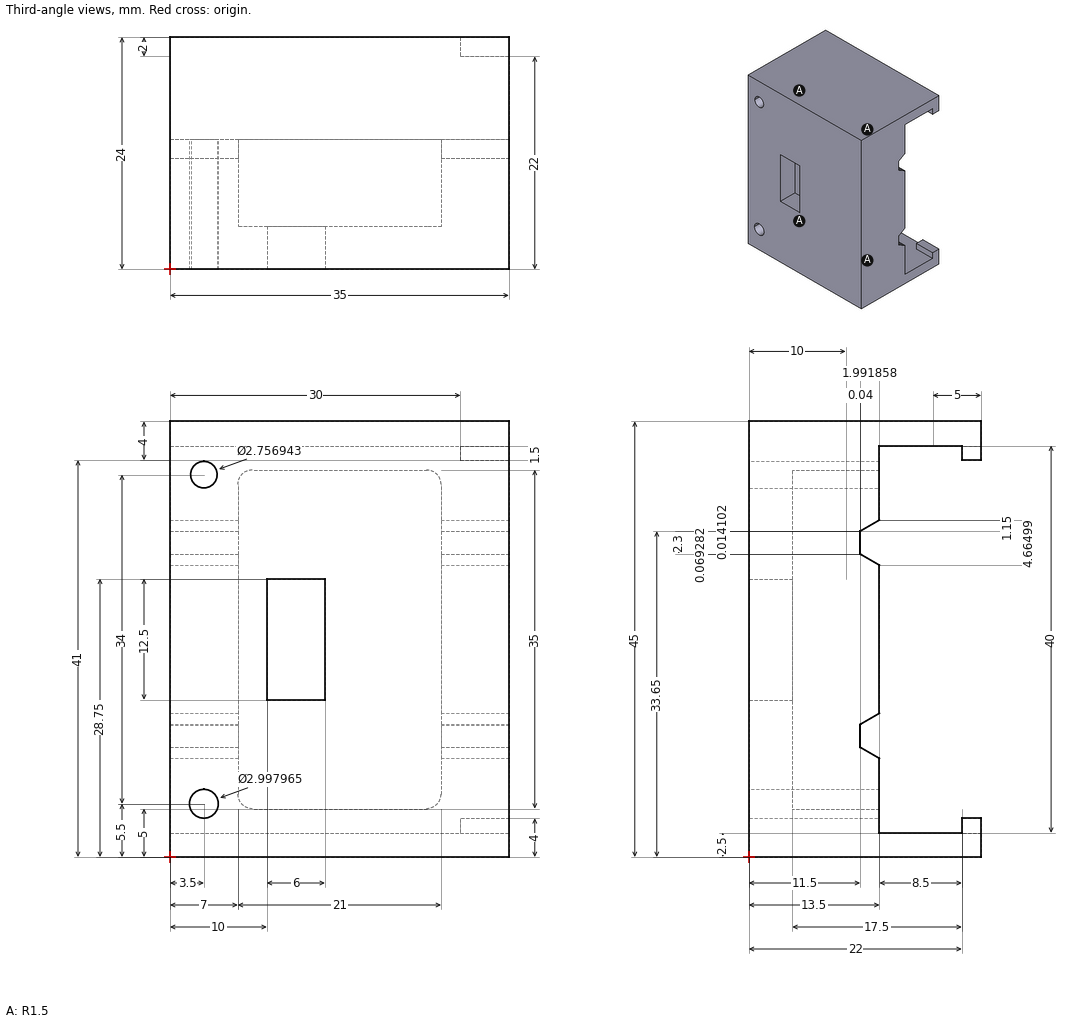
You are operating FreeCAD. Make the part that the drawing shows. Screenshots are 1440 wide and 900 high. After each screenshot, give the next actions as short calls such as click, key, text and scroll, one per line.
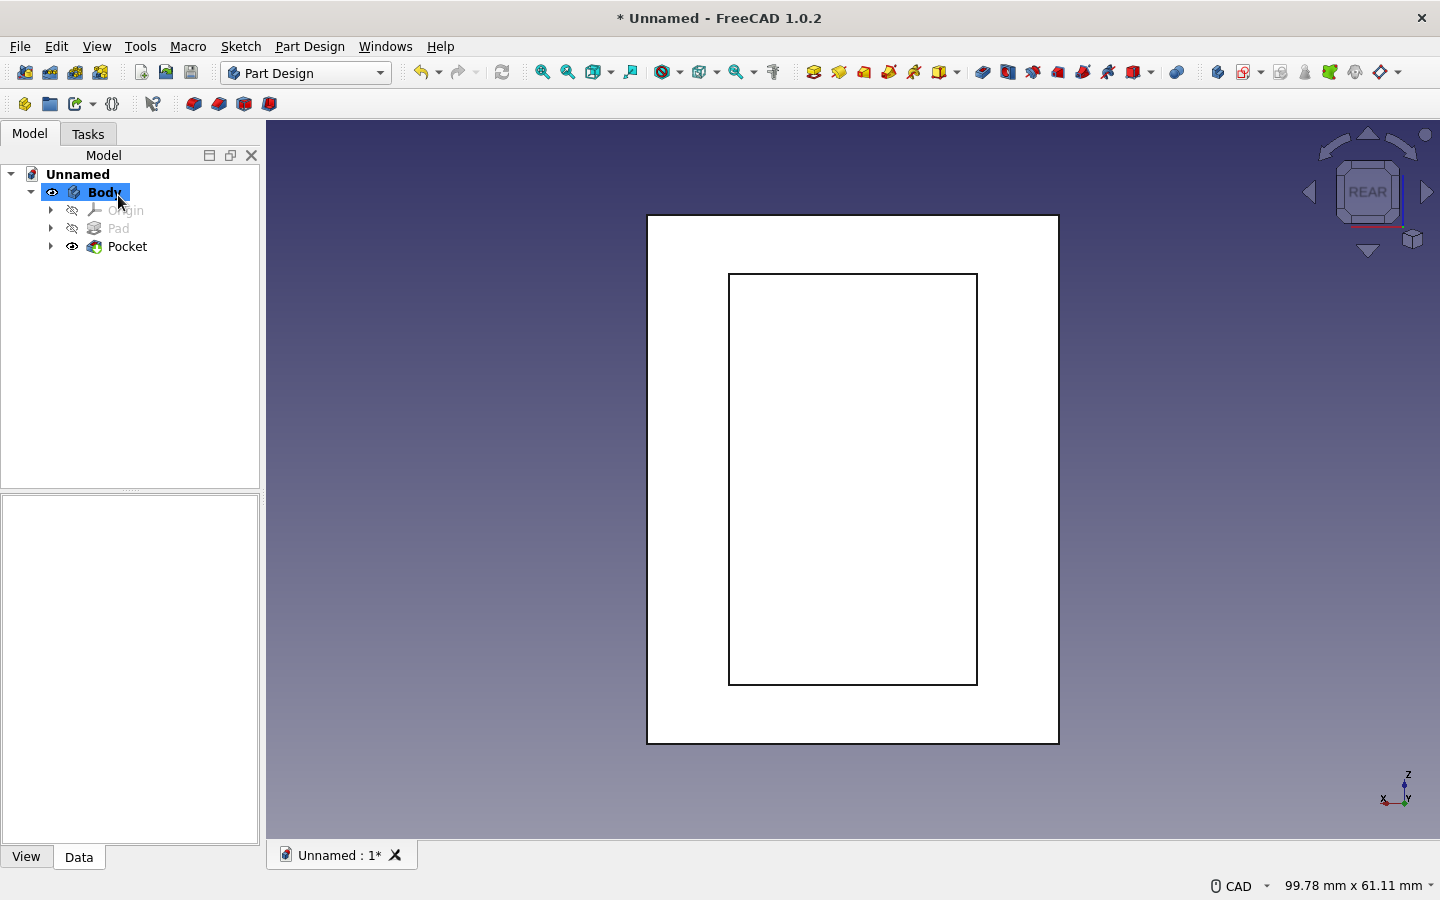
click(1242, 72)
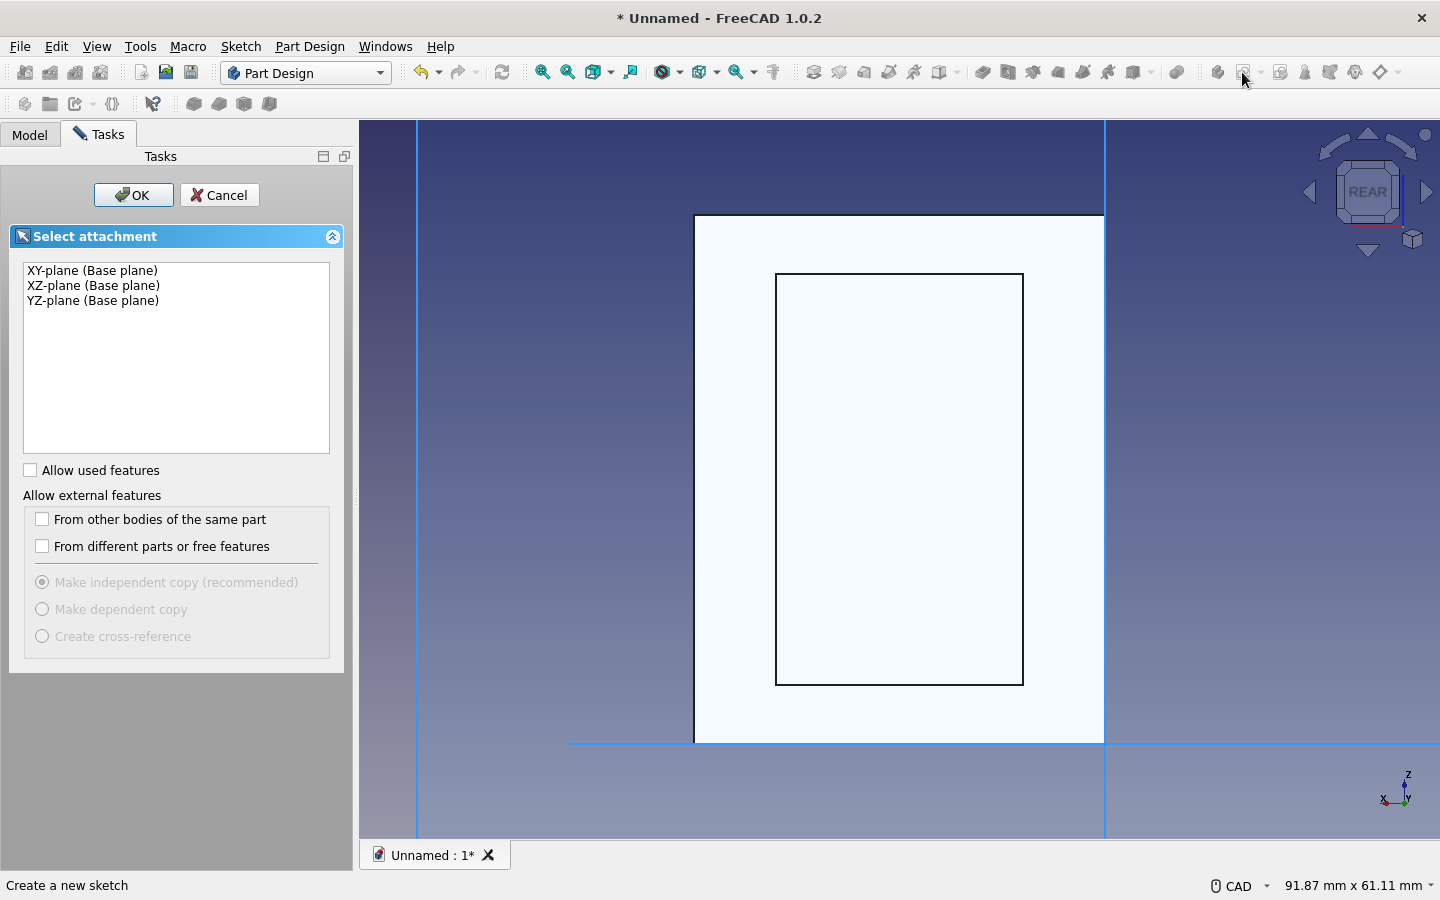
click(84, 300)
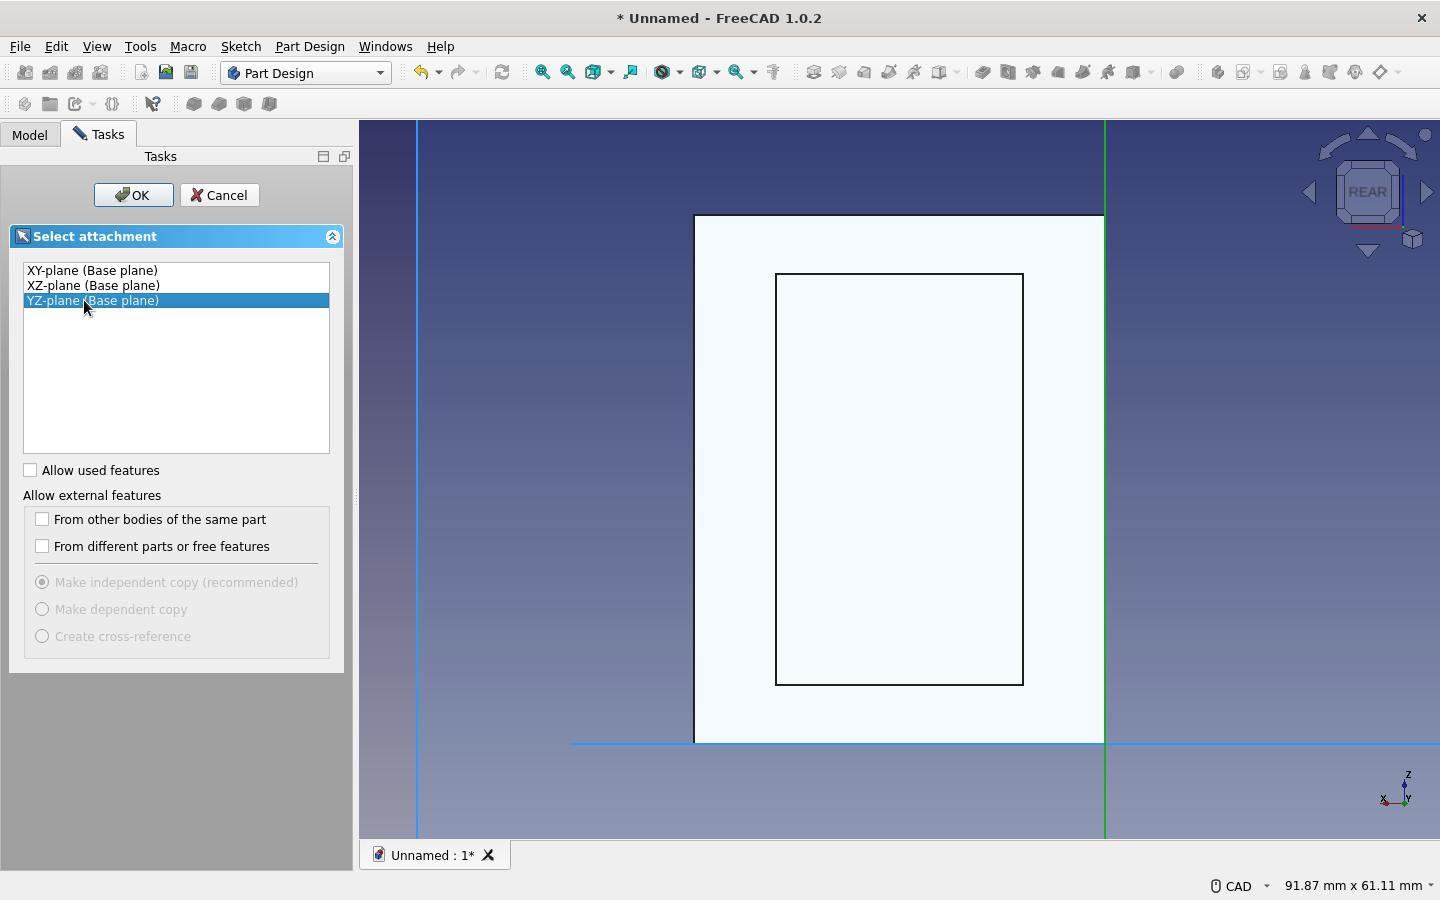
click(134, 195)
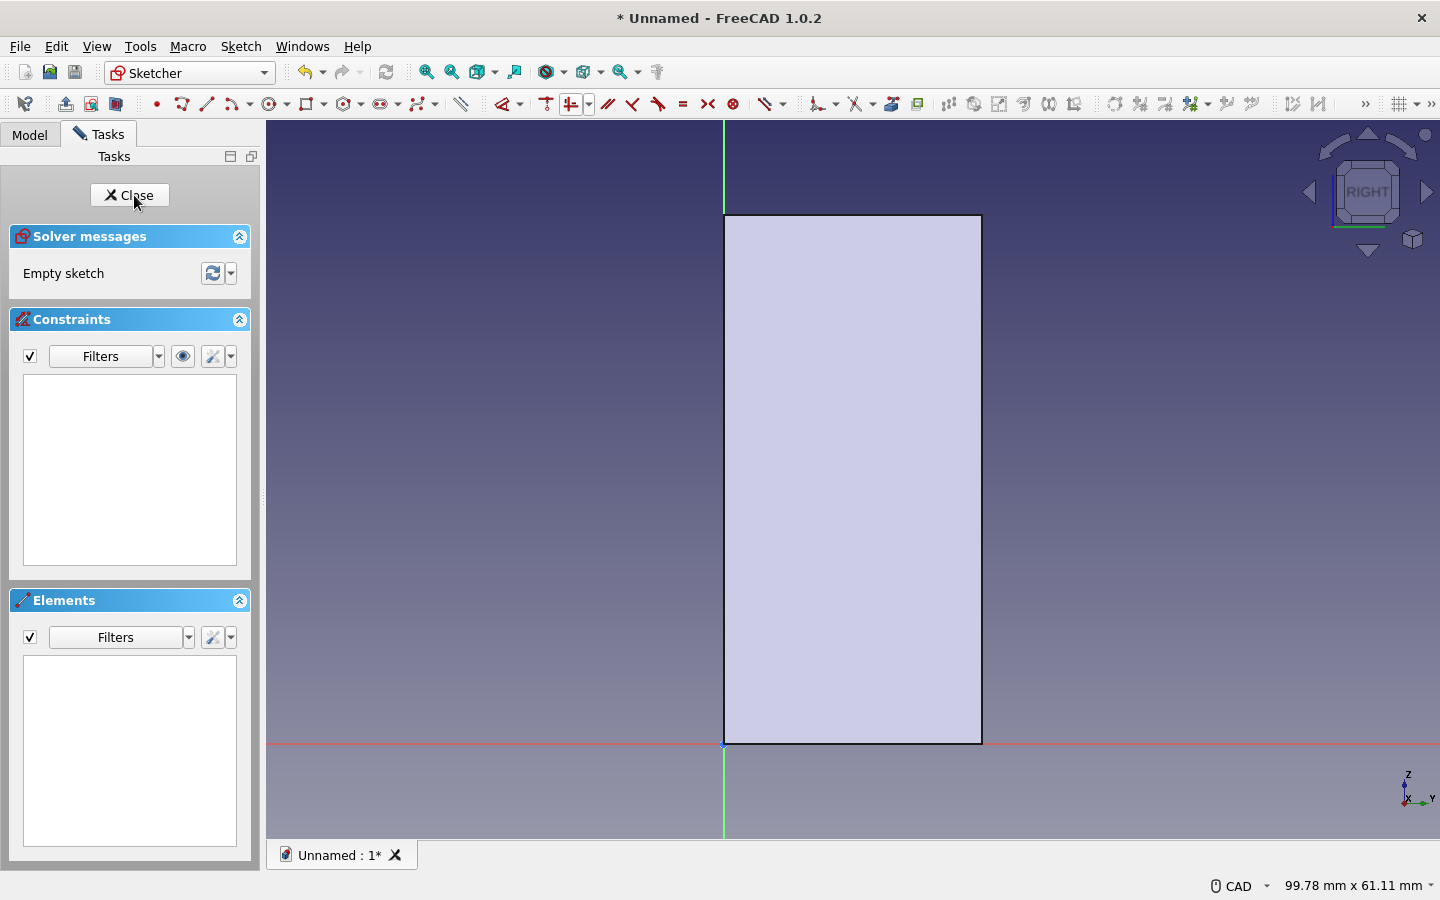
click(116, 104)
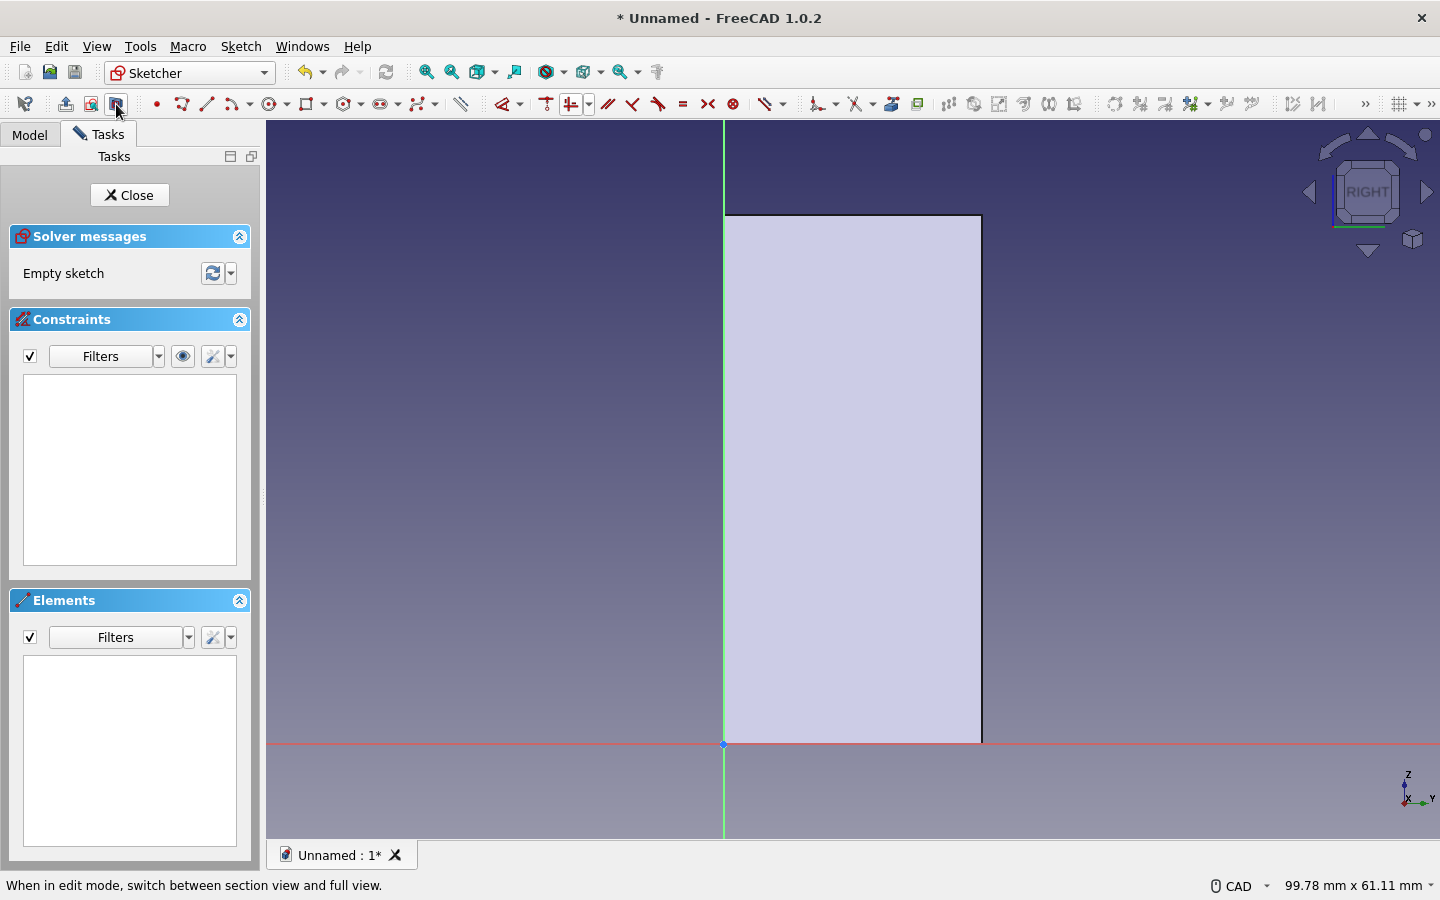
click(306, 104)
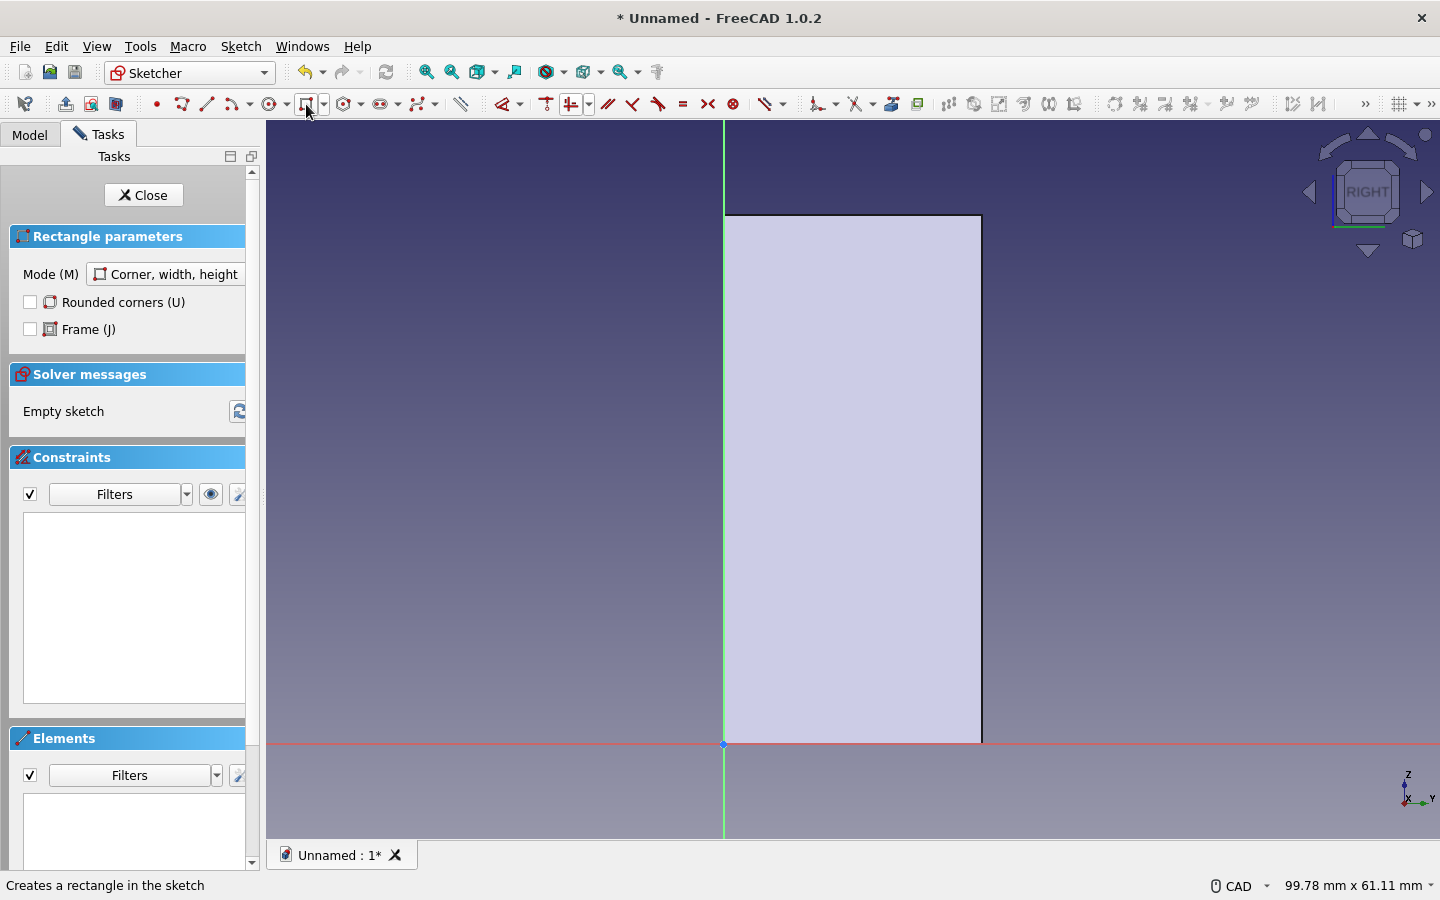
click(882, 244)
click(982, 715)
key(Escape)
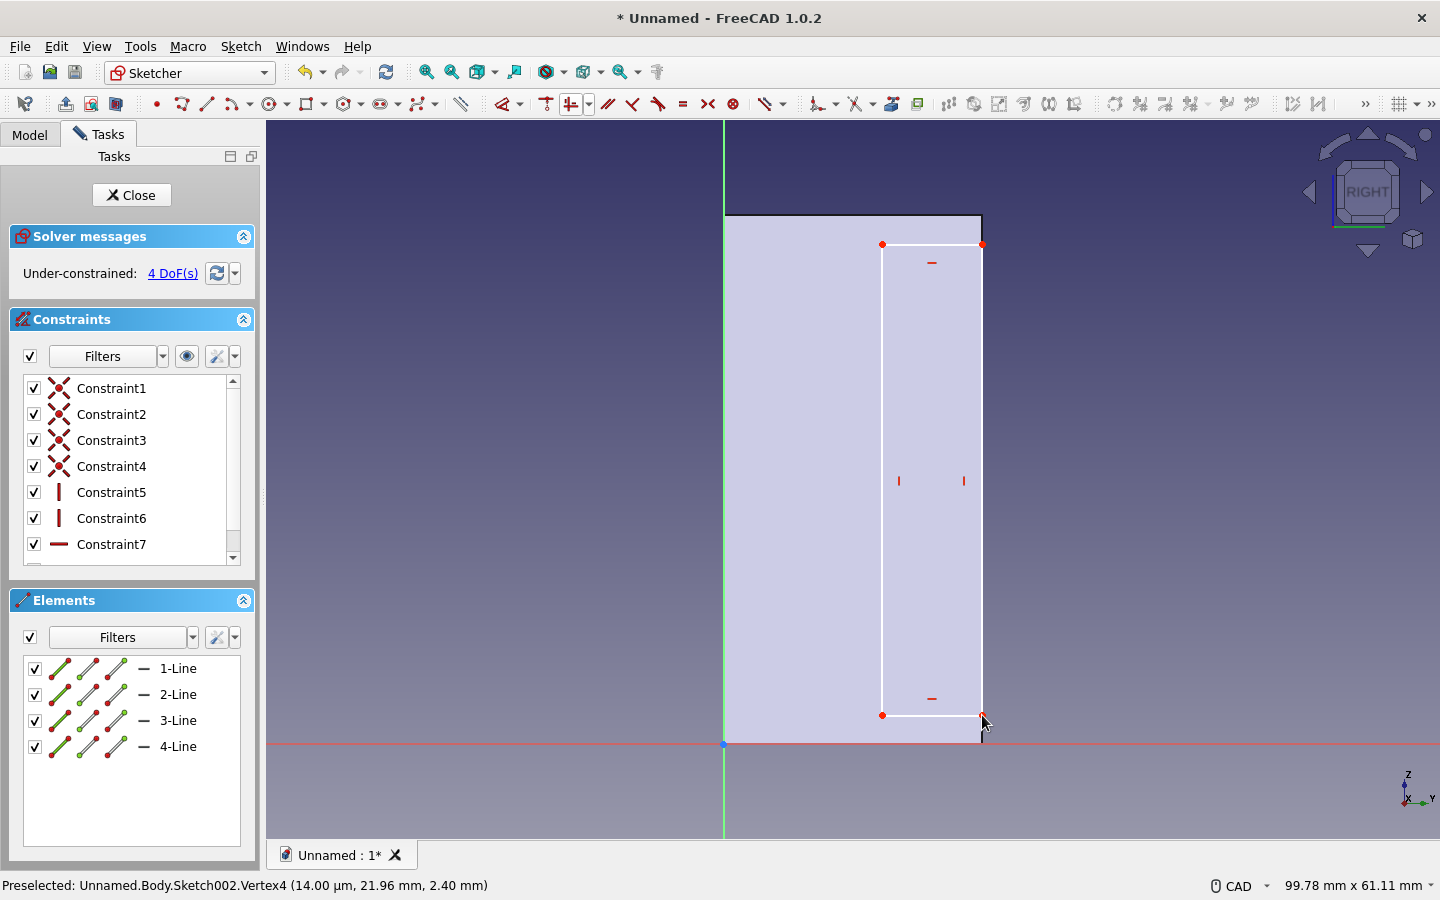
click(502, 104)